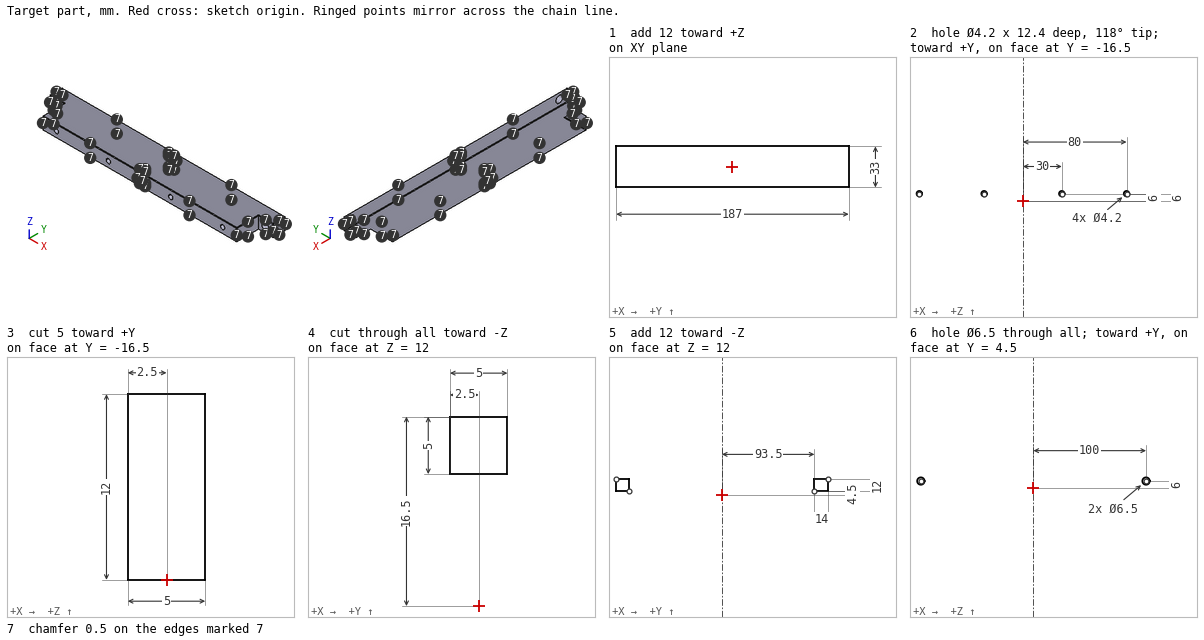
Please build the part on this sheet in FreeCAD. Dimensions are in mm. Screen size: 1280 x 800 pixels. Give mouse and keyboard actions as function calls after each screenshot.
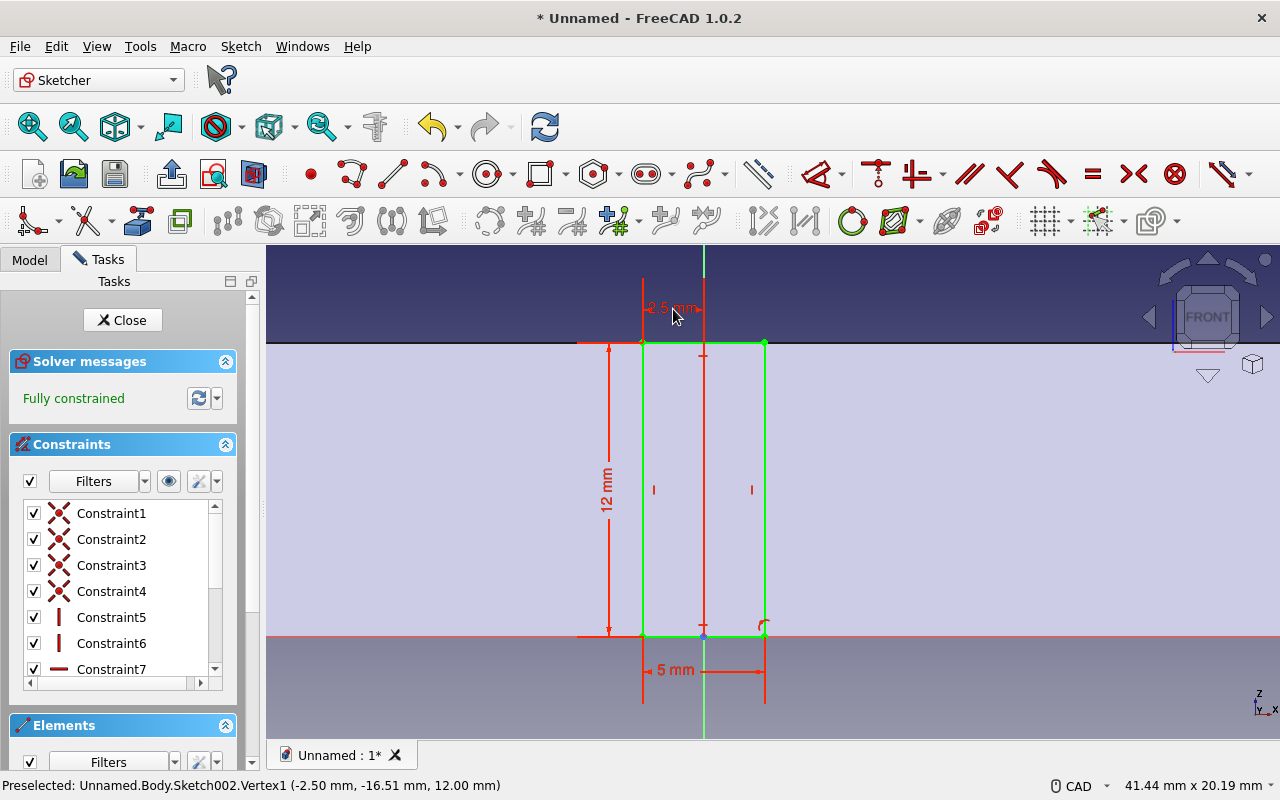
click(123, 320)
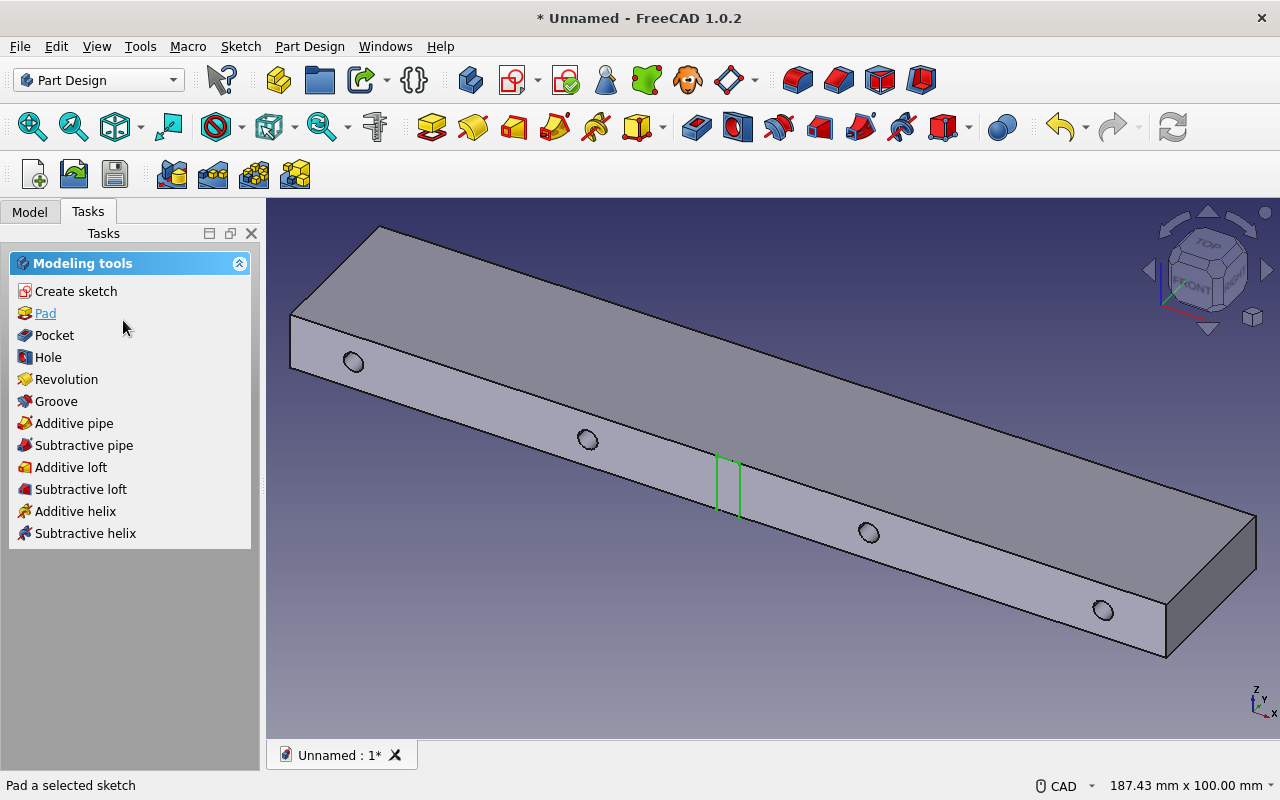
click(697, 128)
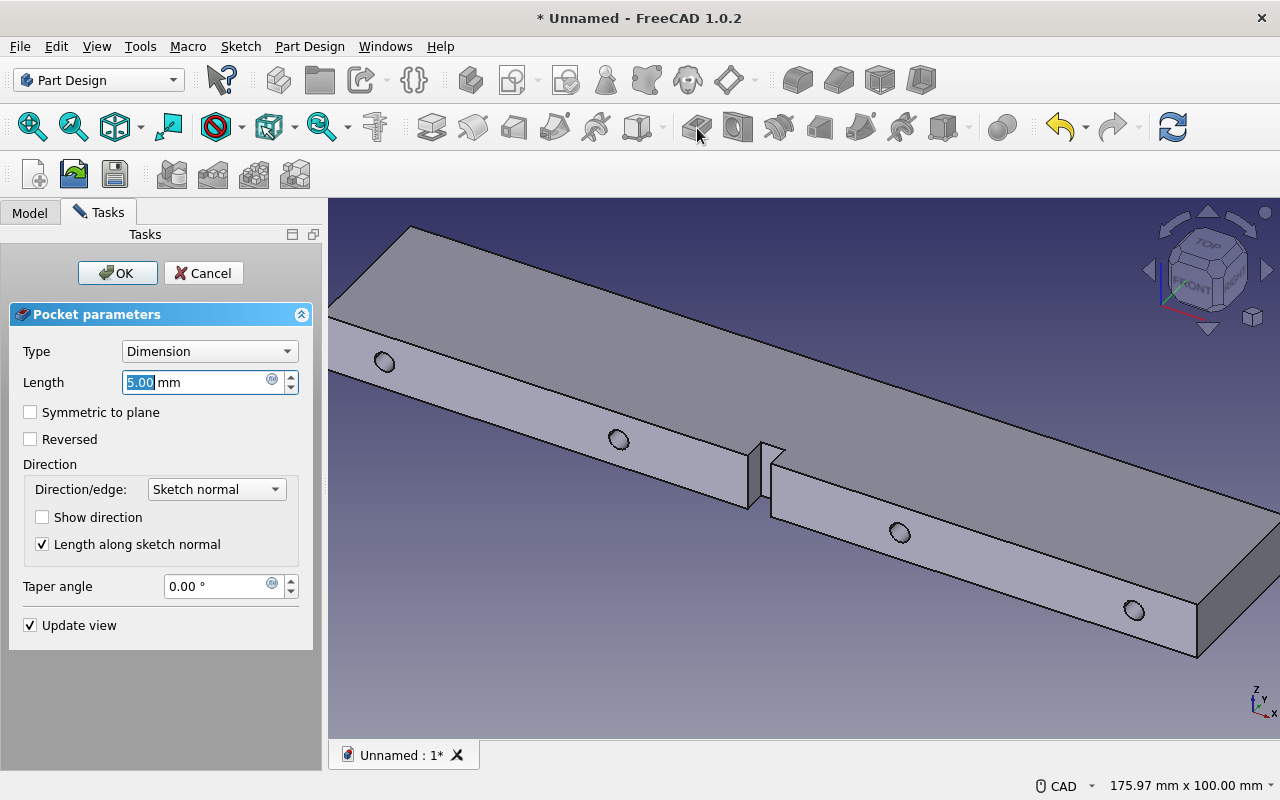
text(5)
key(Tab)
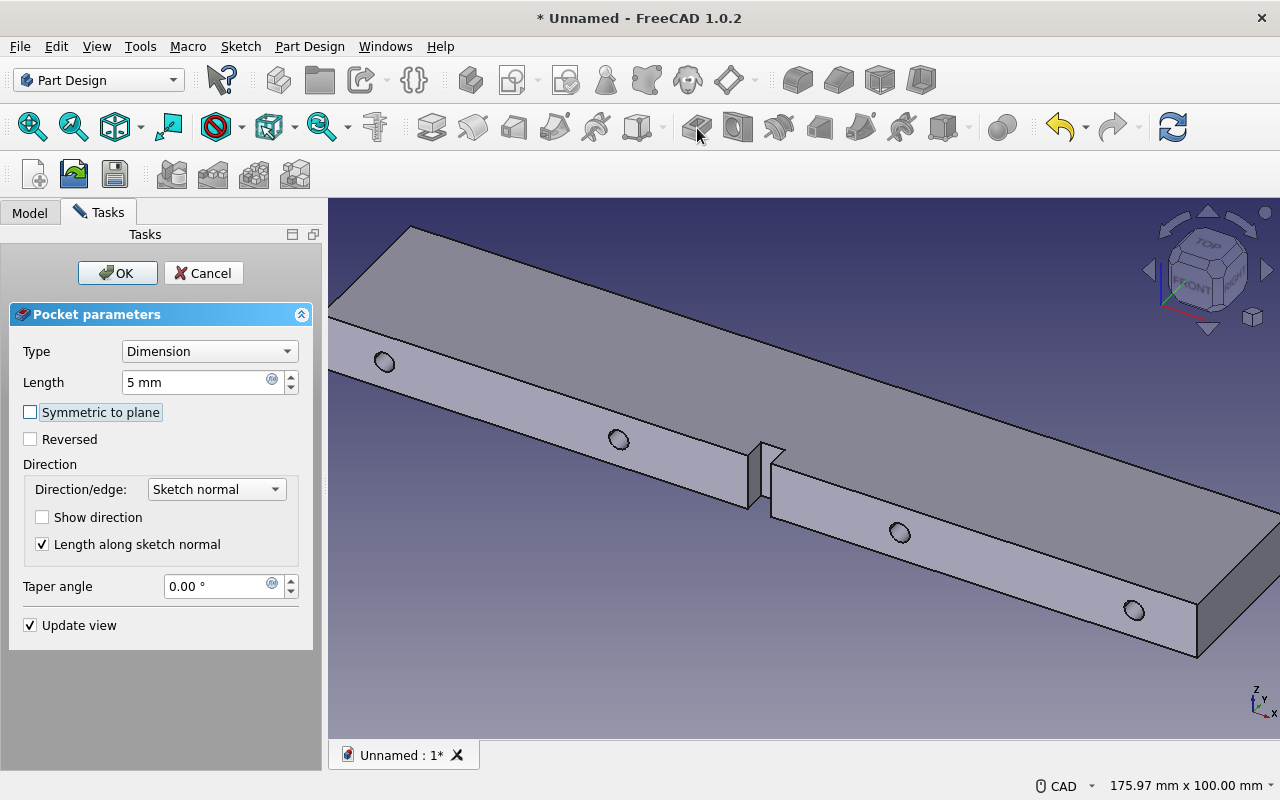
click(118, 273)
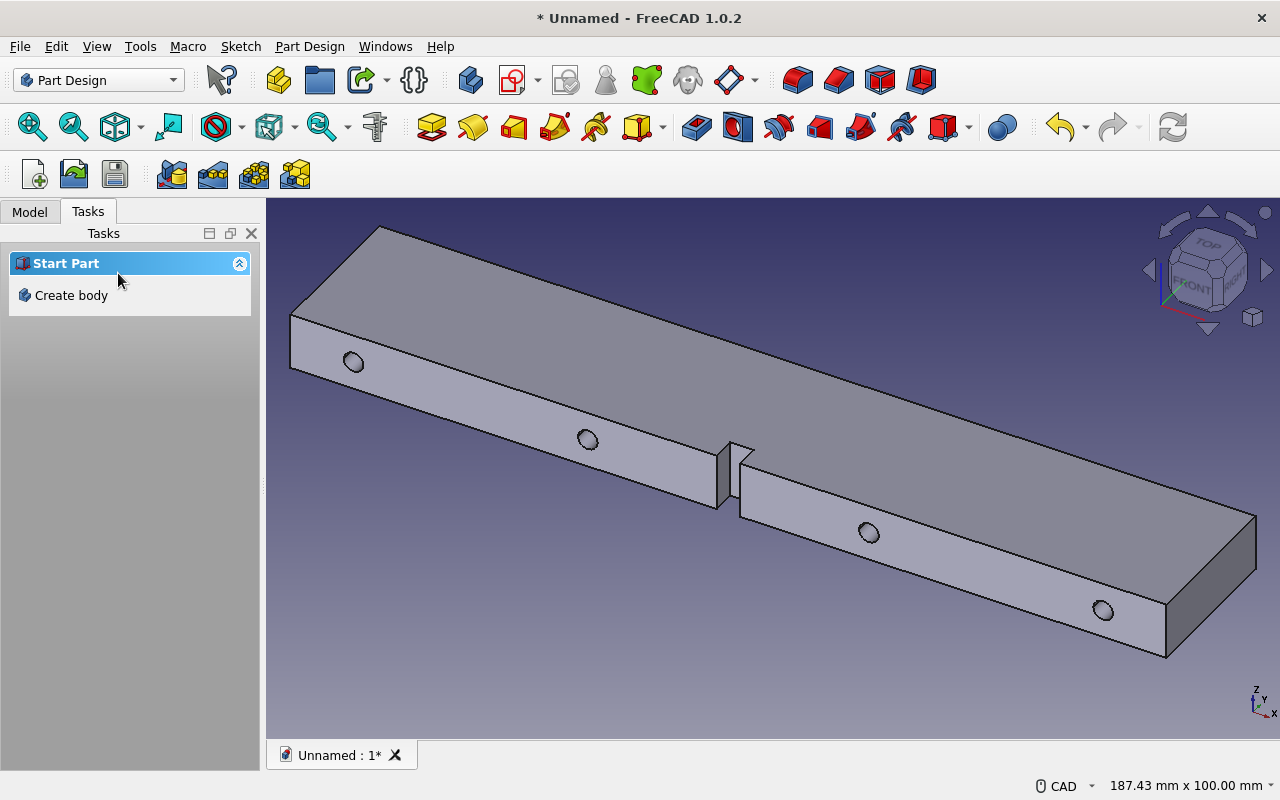
click(1023, 497)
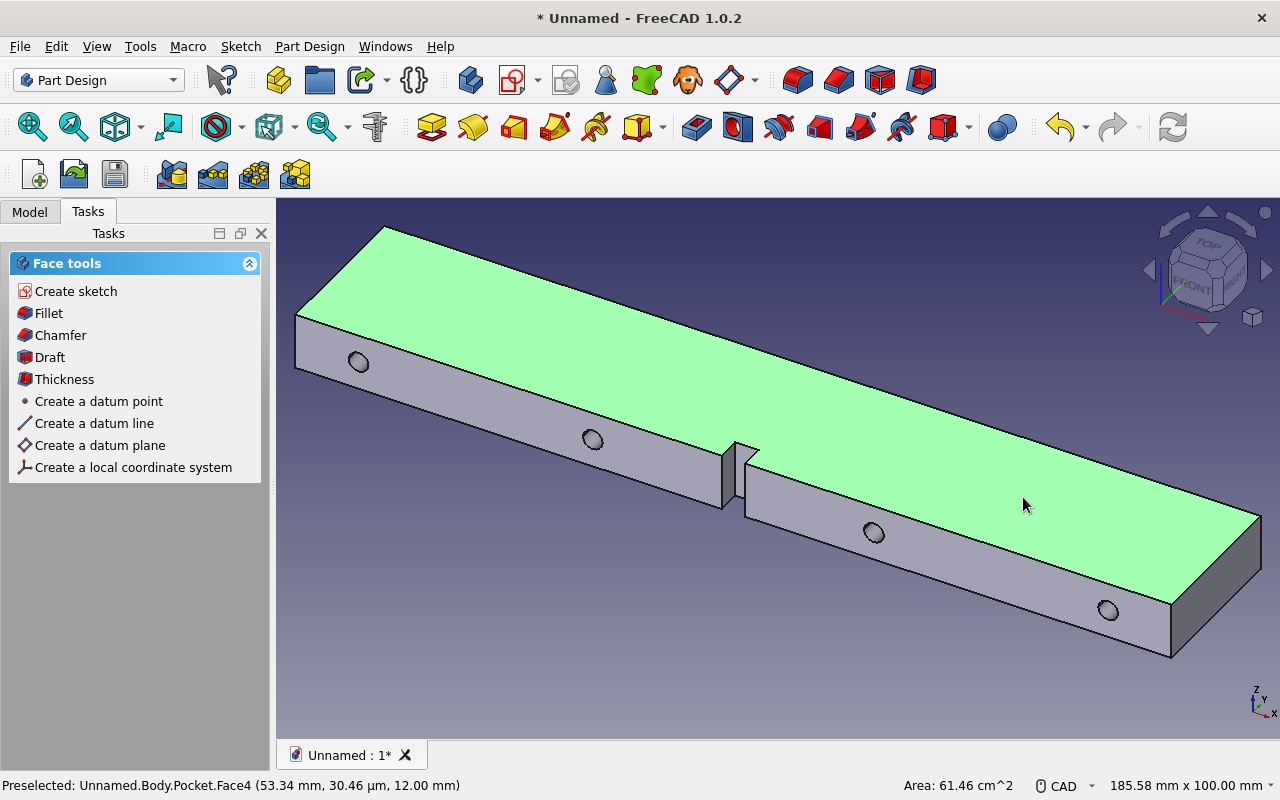
click(512, 80)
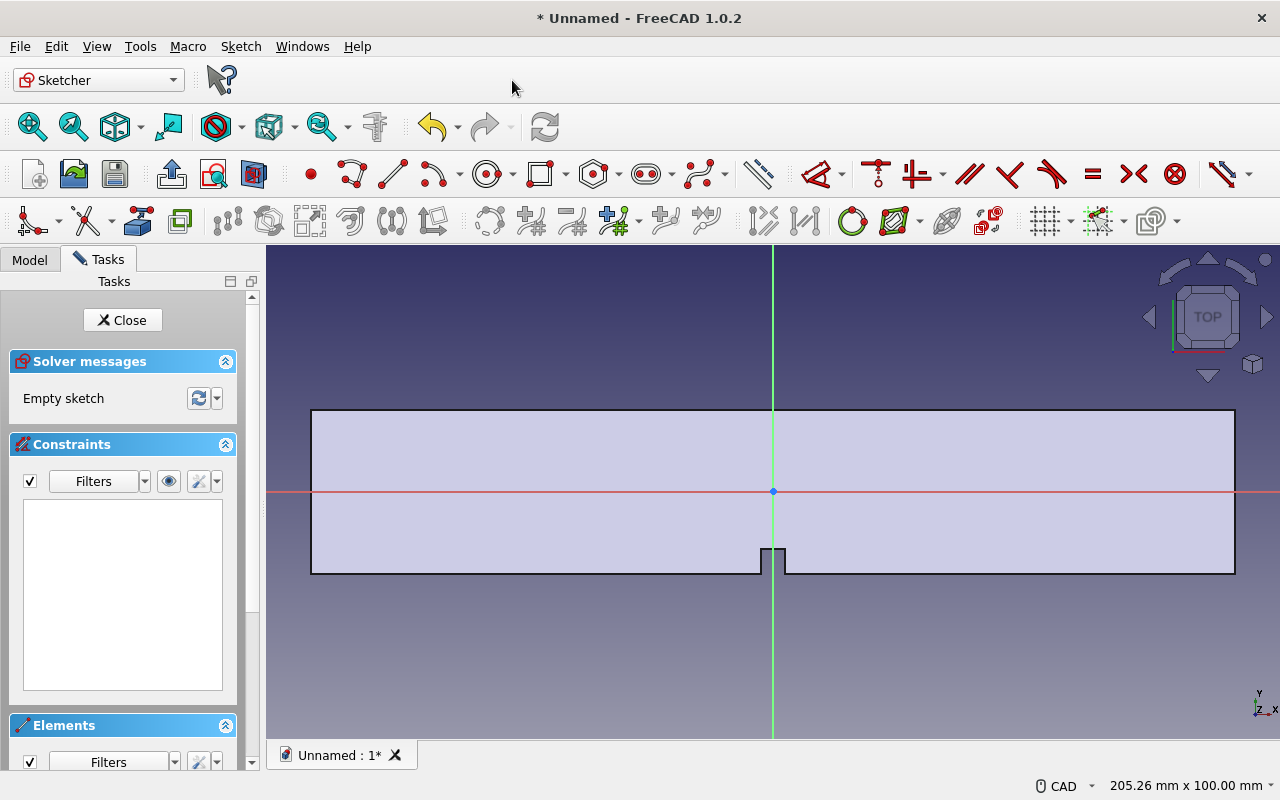
scroll(778, 417, up, 13)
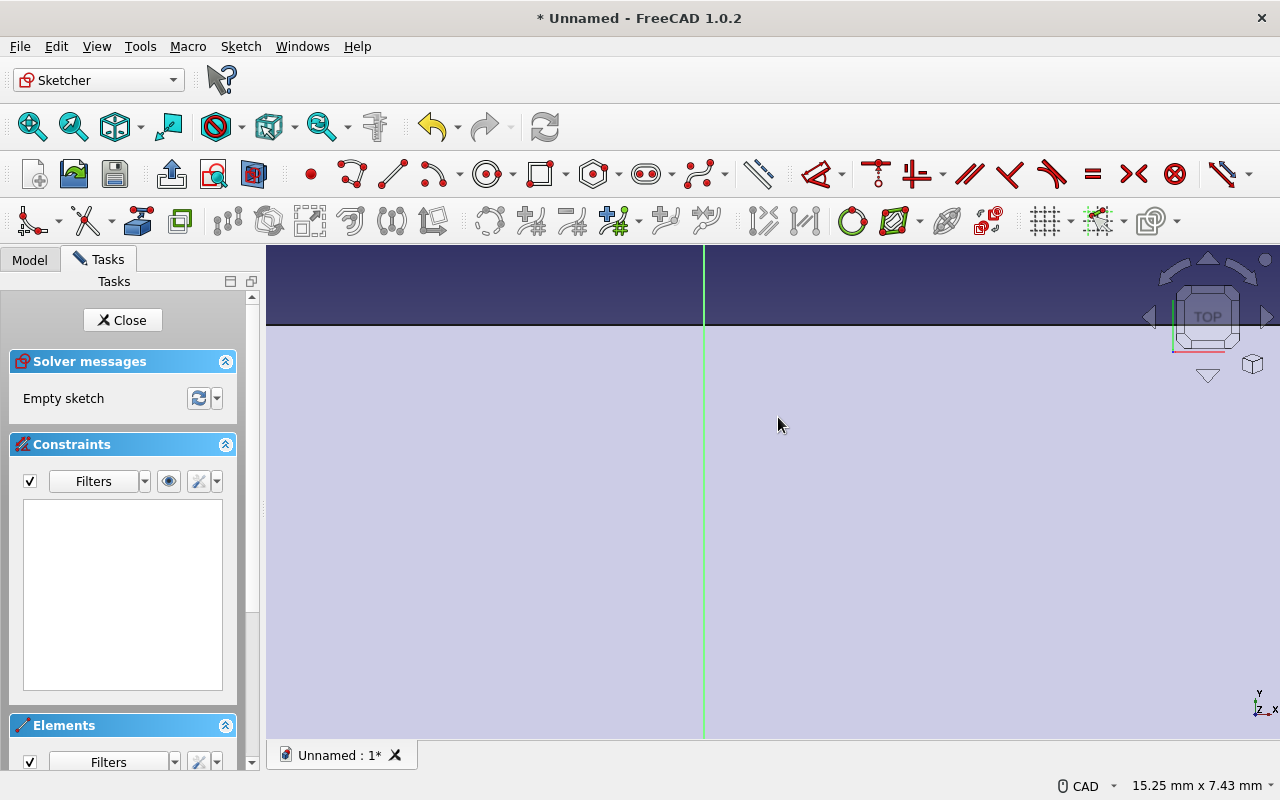
key(g)
key(r)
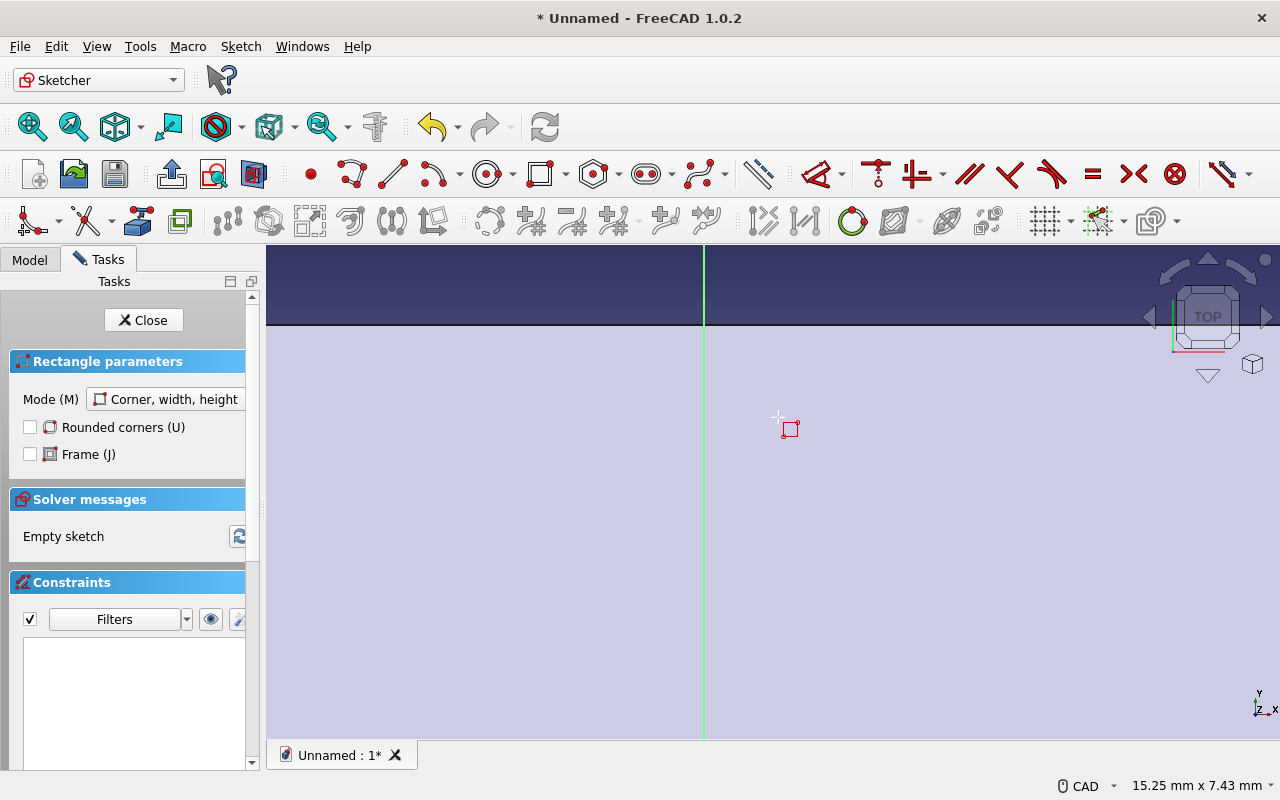
click(538, 325)
click(871, 658)
key(Escape)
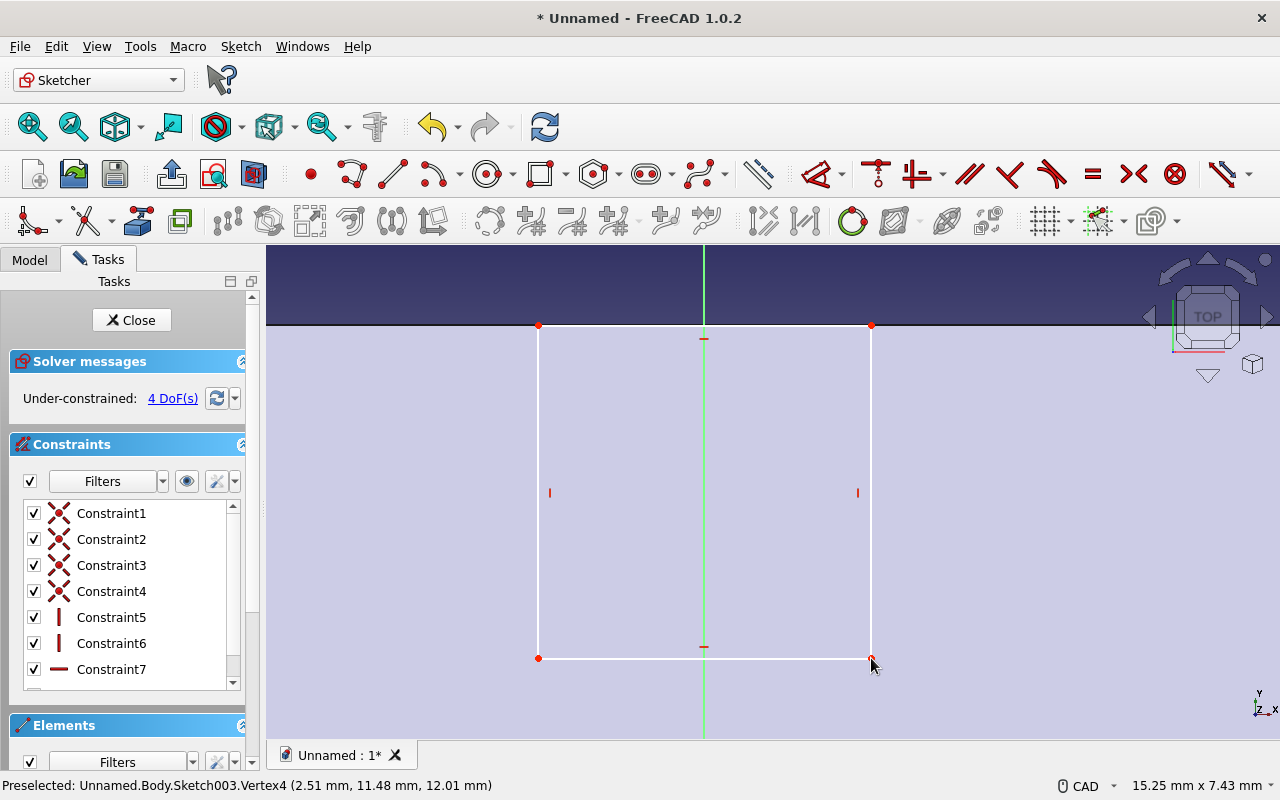
click(816, 174)